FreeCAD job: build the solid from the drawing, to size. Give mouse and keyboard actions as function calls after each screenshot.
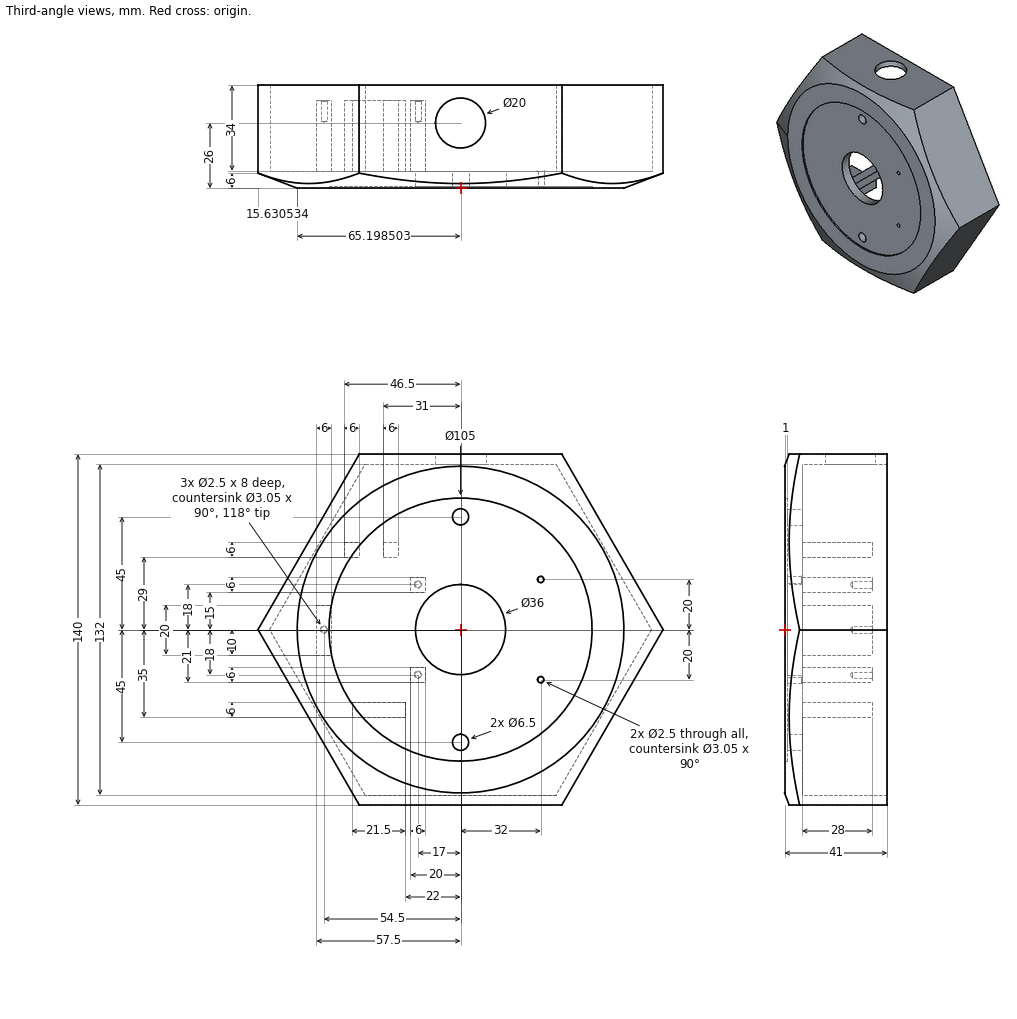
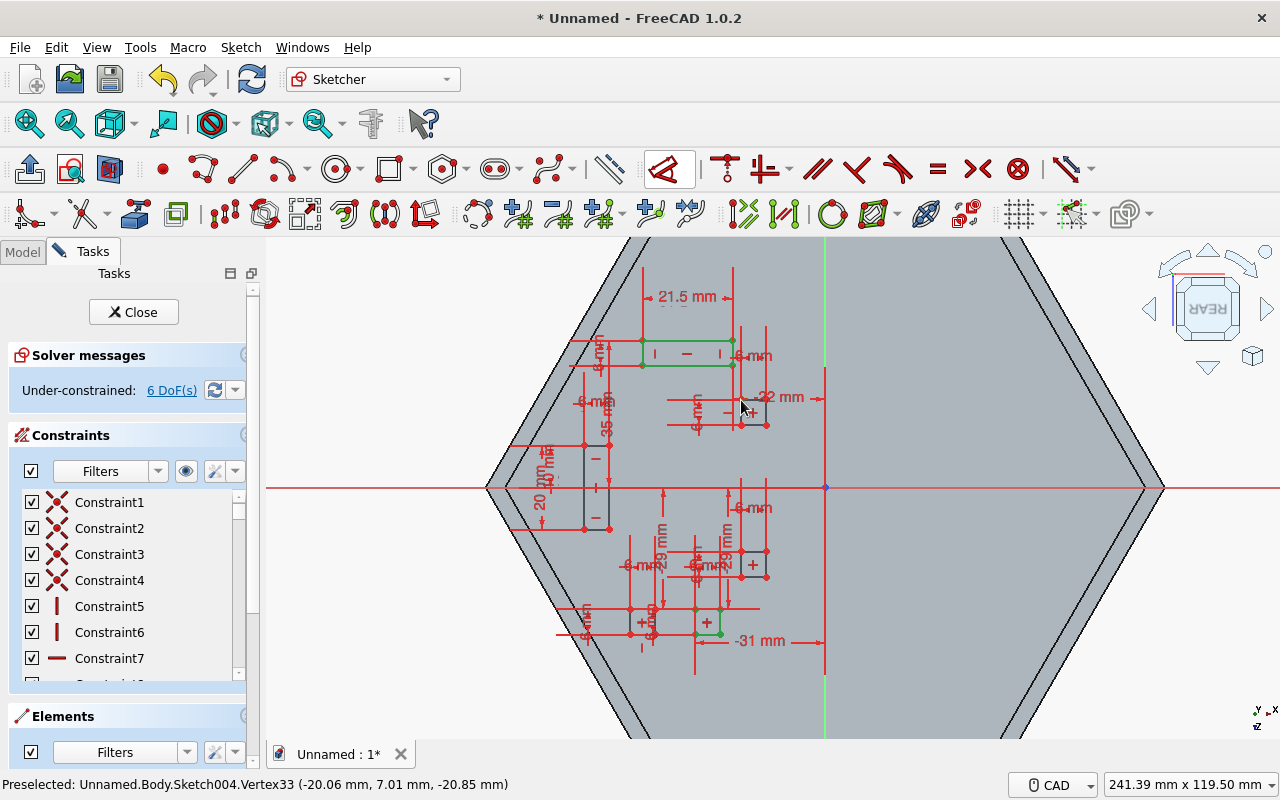
key(l)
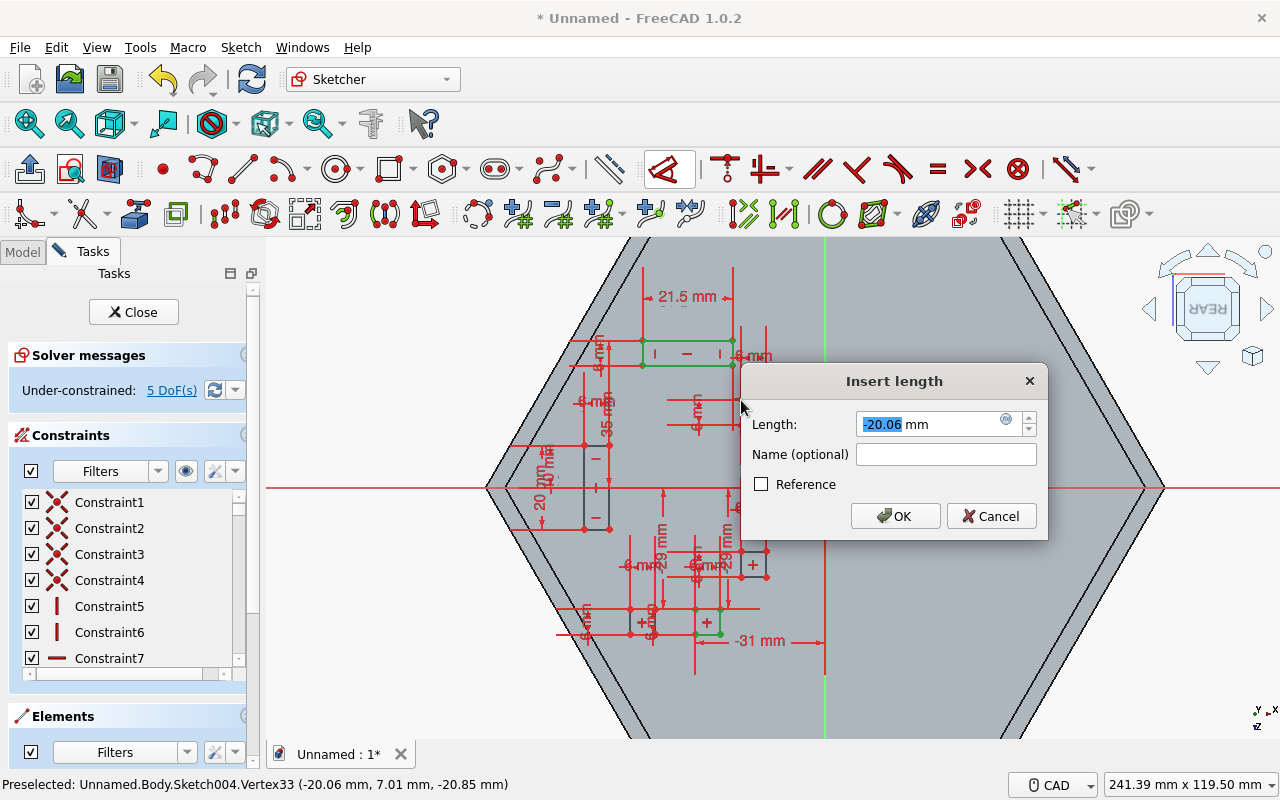
text(-20)
key(Return)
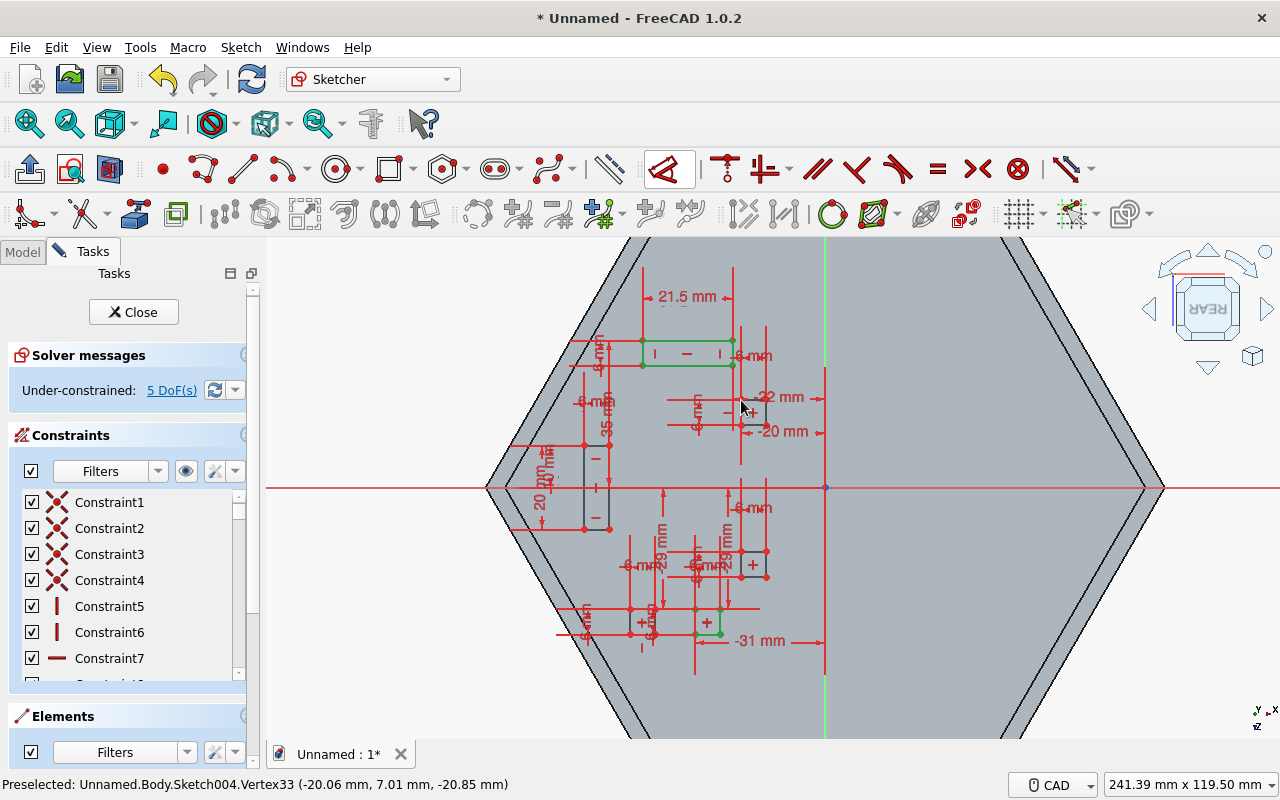
click(741, 400)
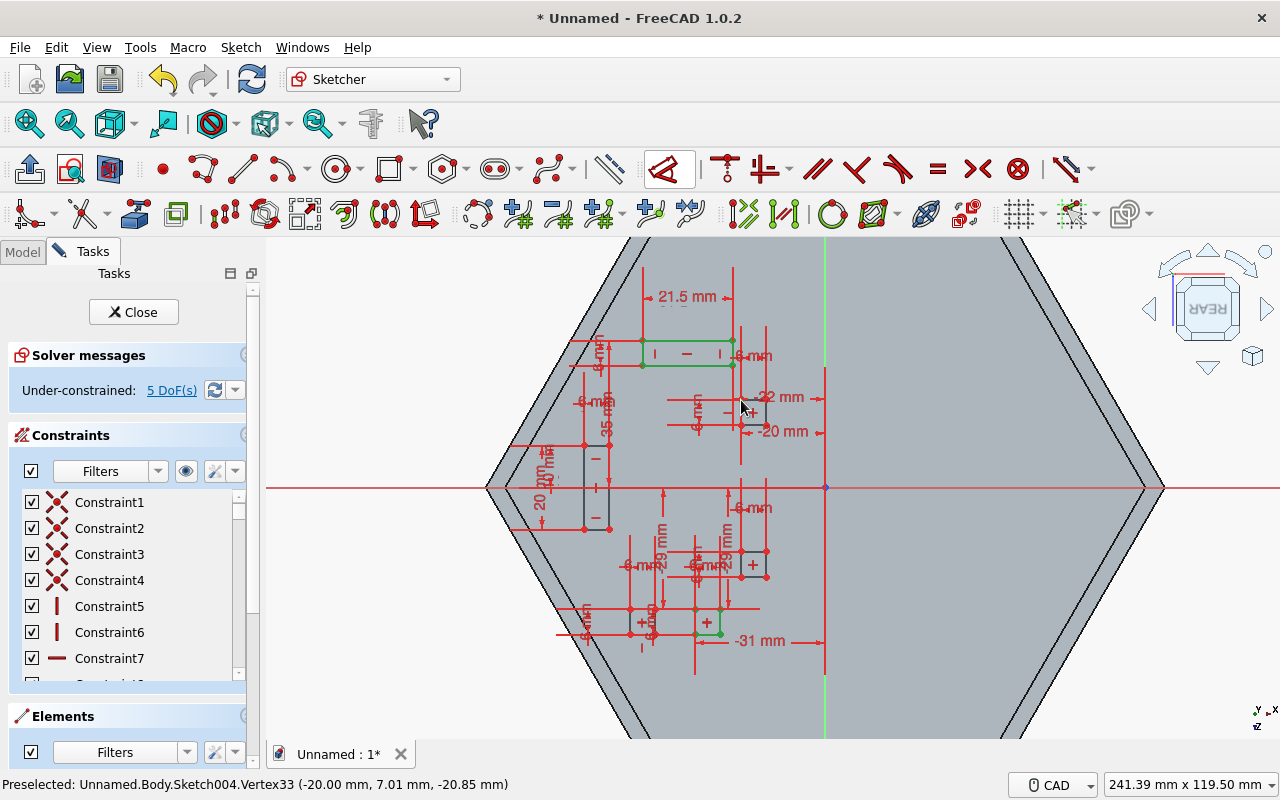
key(i)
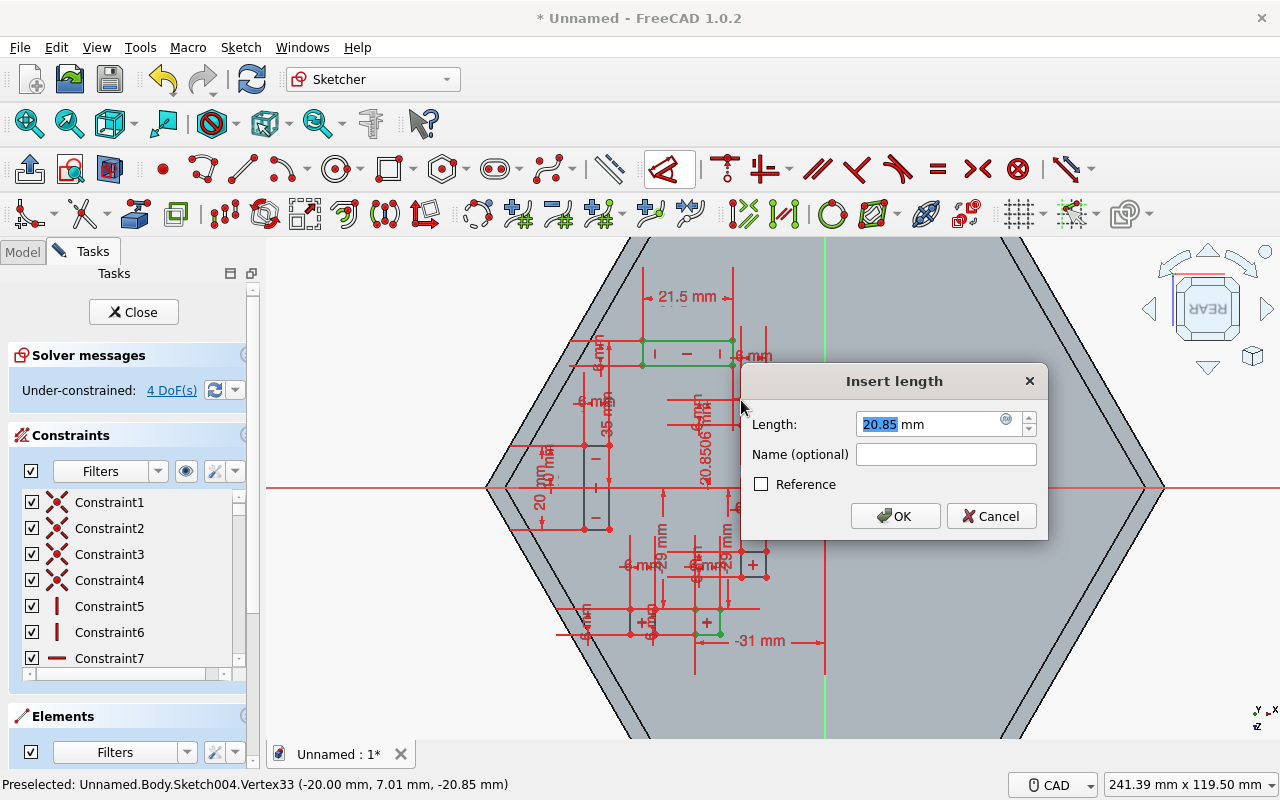
text(21)
key(Return)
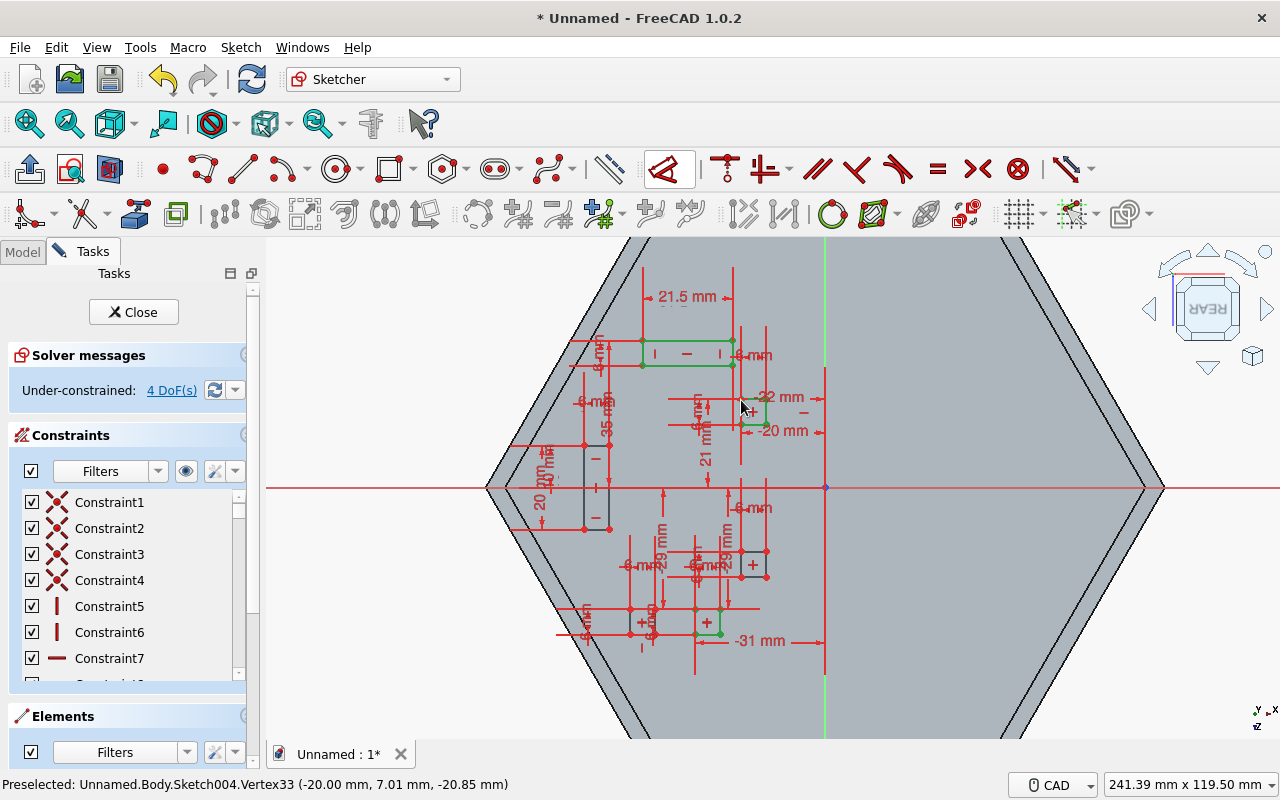
click(741, 552)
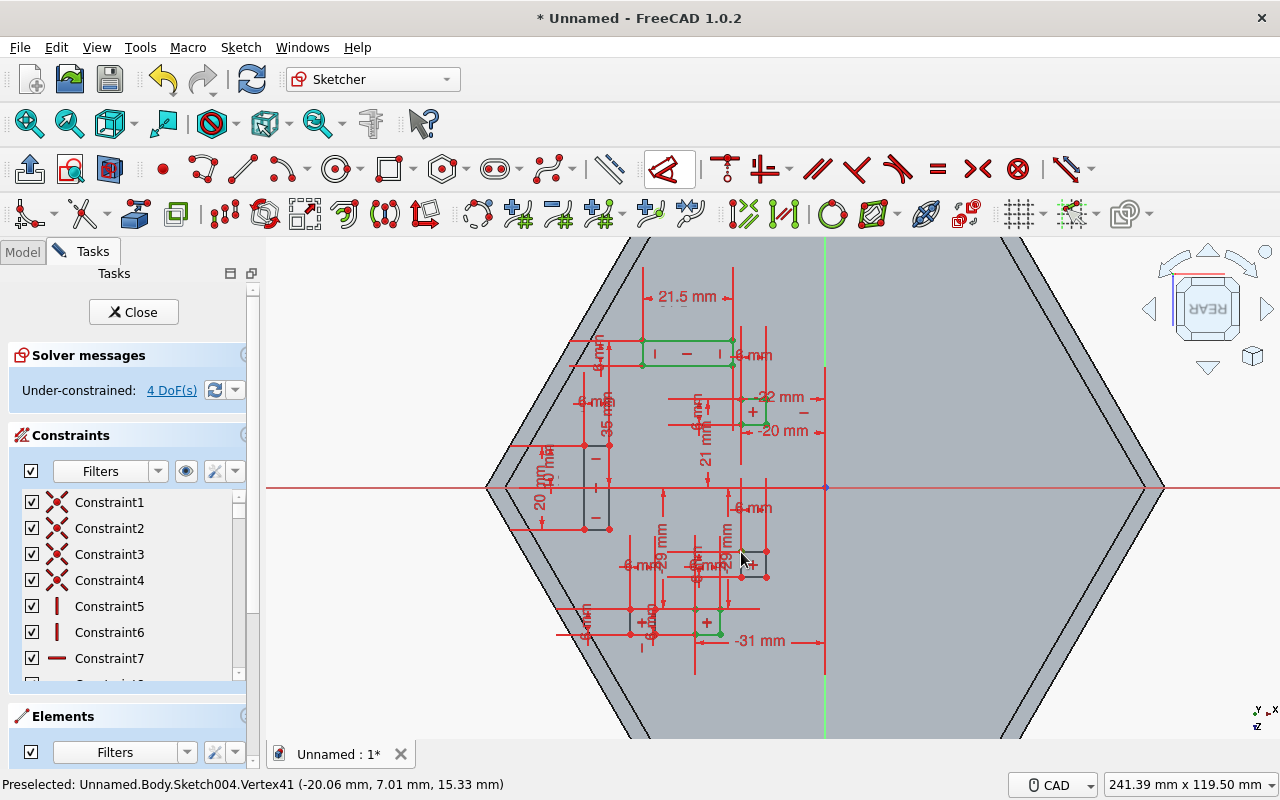
key(l)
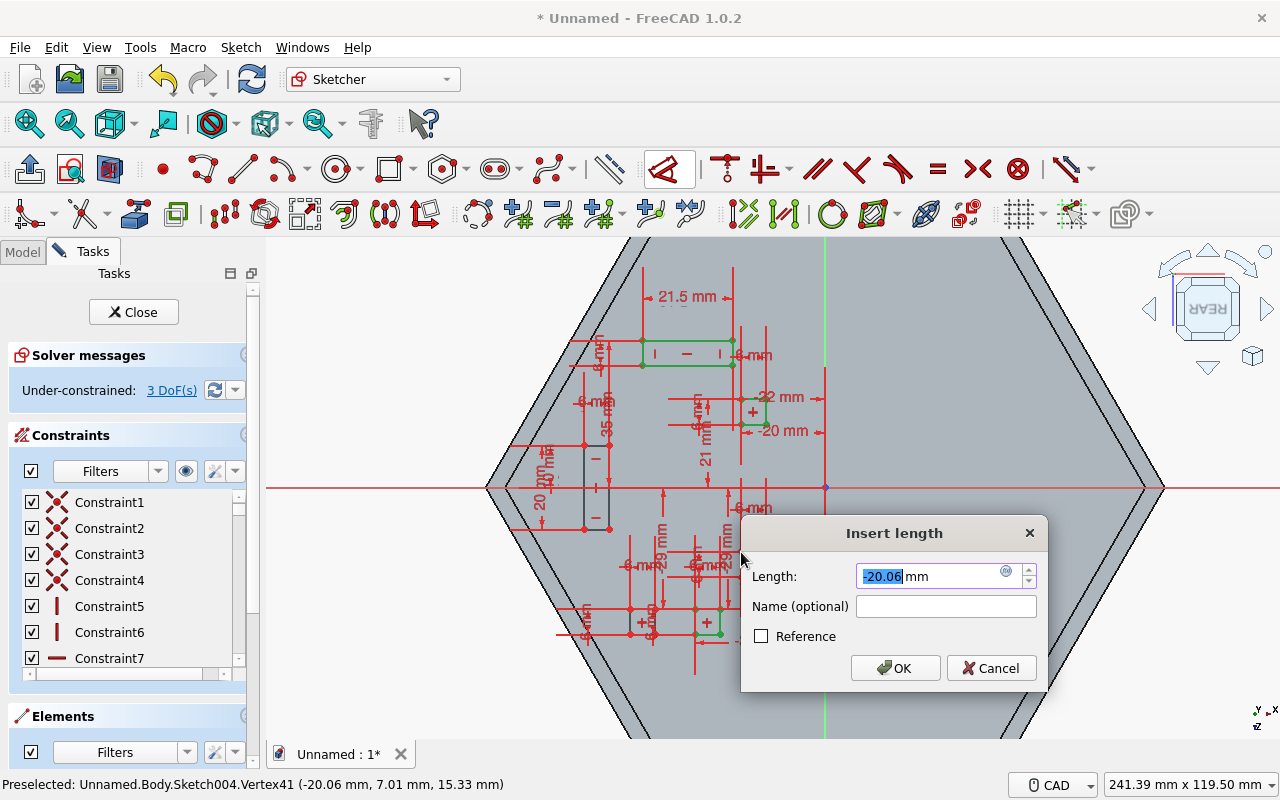
text(-20)
key(Return)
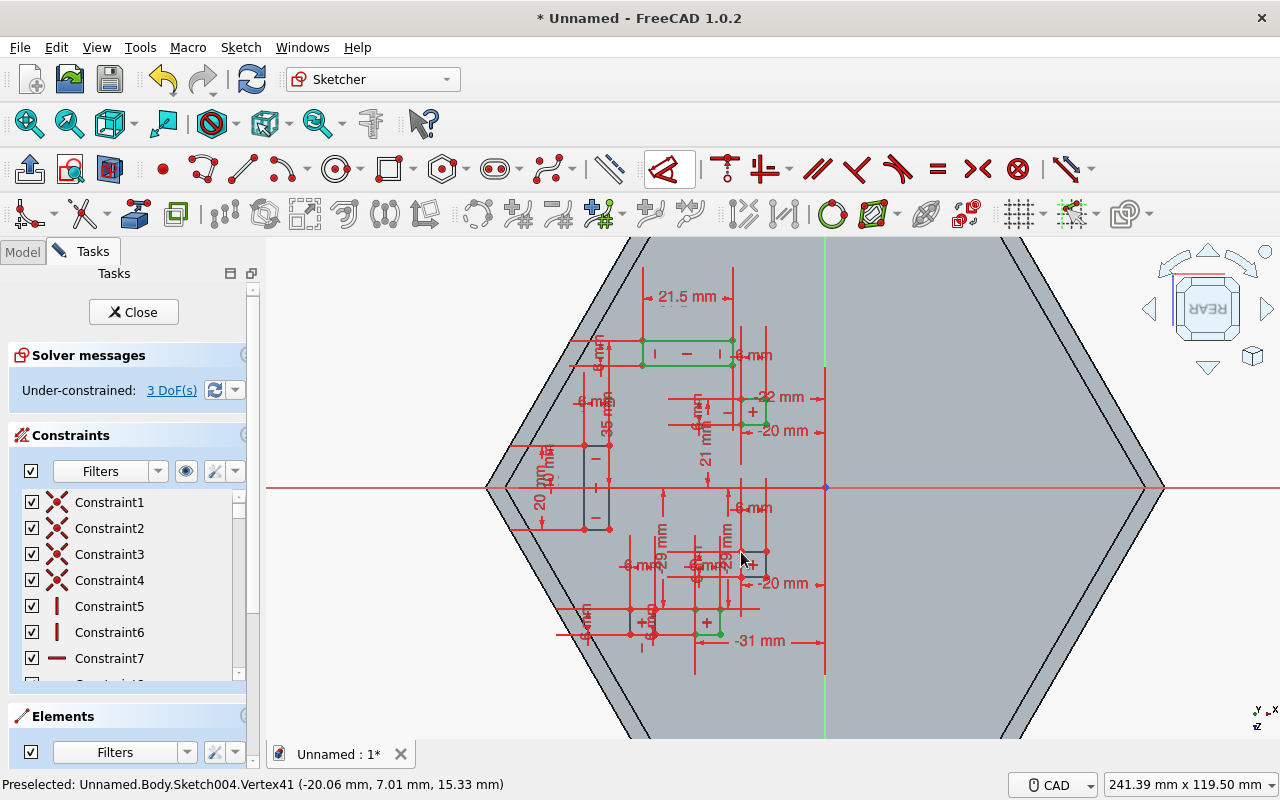
click(741, 552)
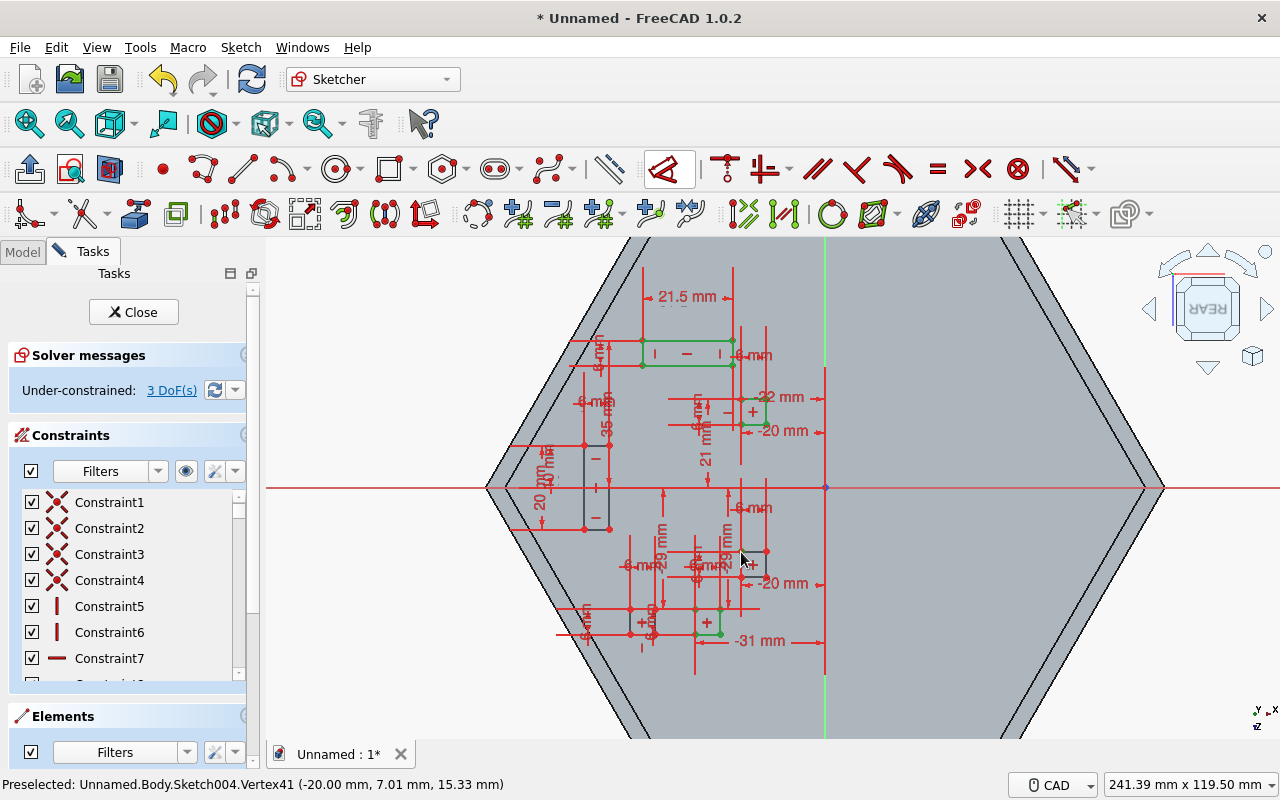
key(i)